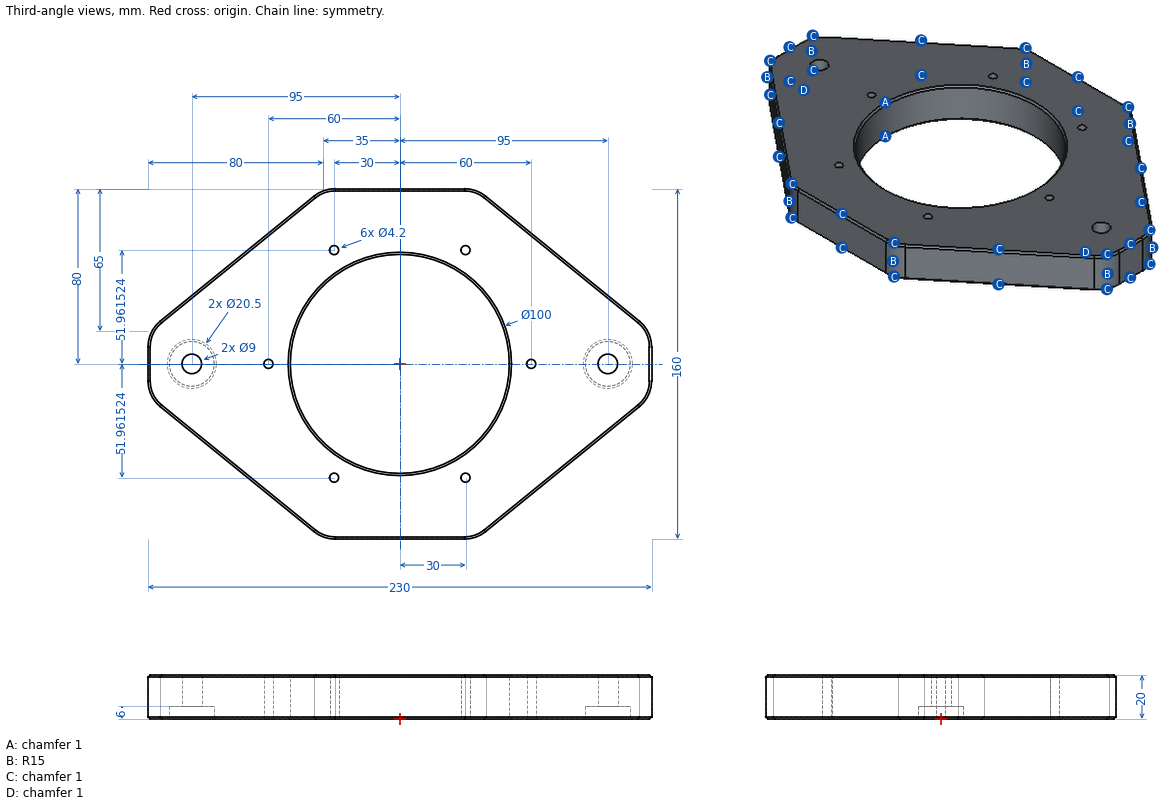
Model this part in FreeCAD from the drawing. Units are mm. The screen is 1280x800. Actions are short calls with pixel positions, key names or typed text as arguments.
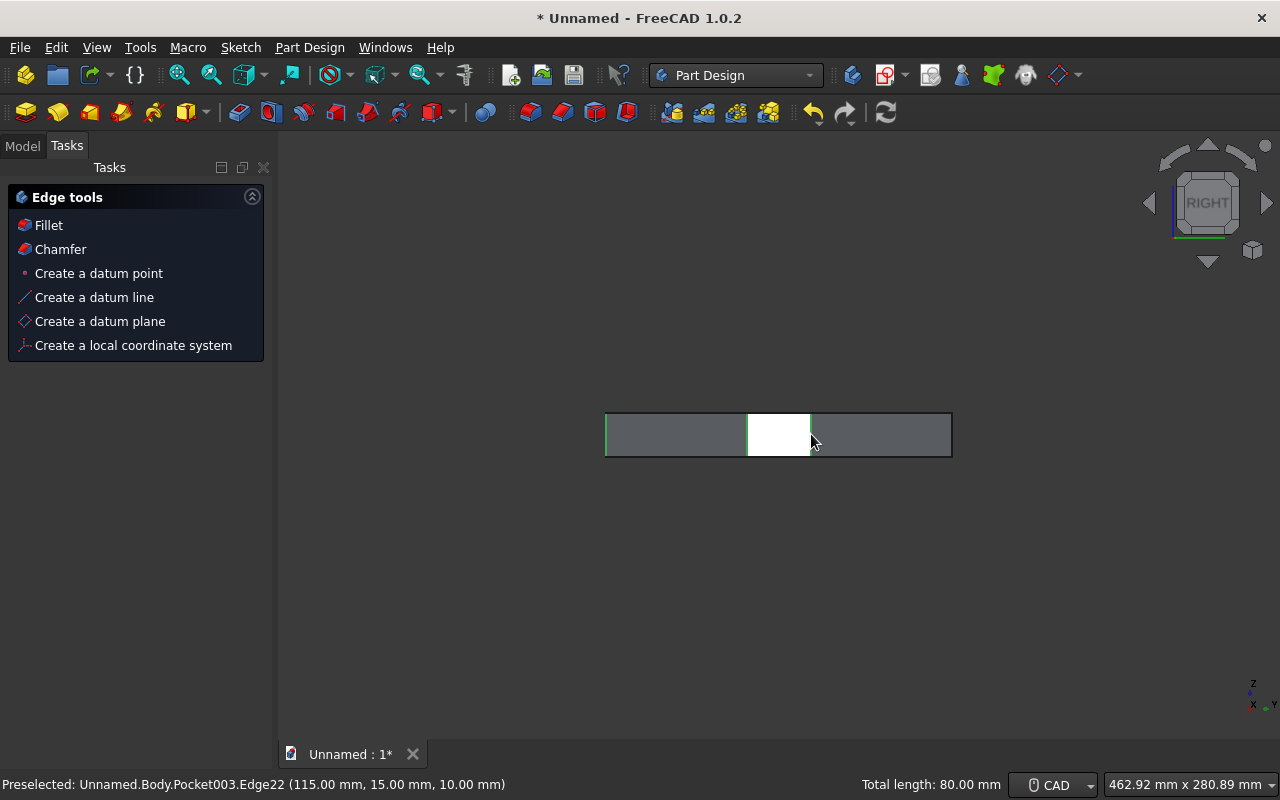
key(5)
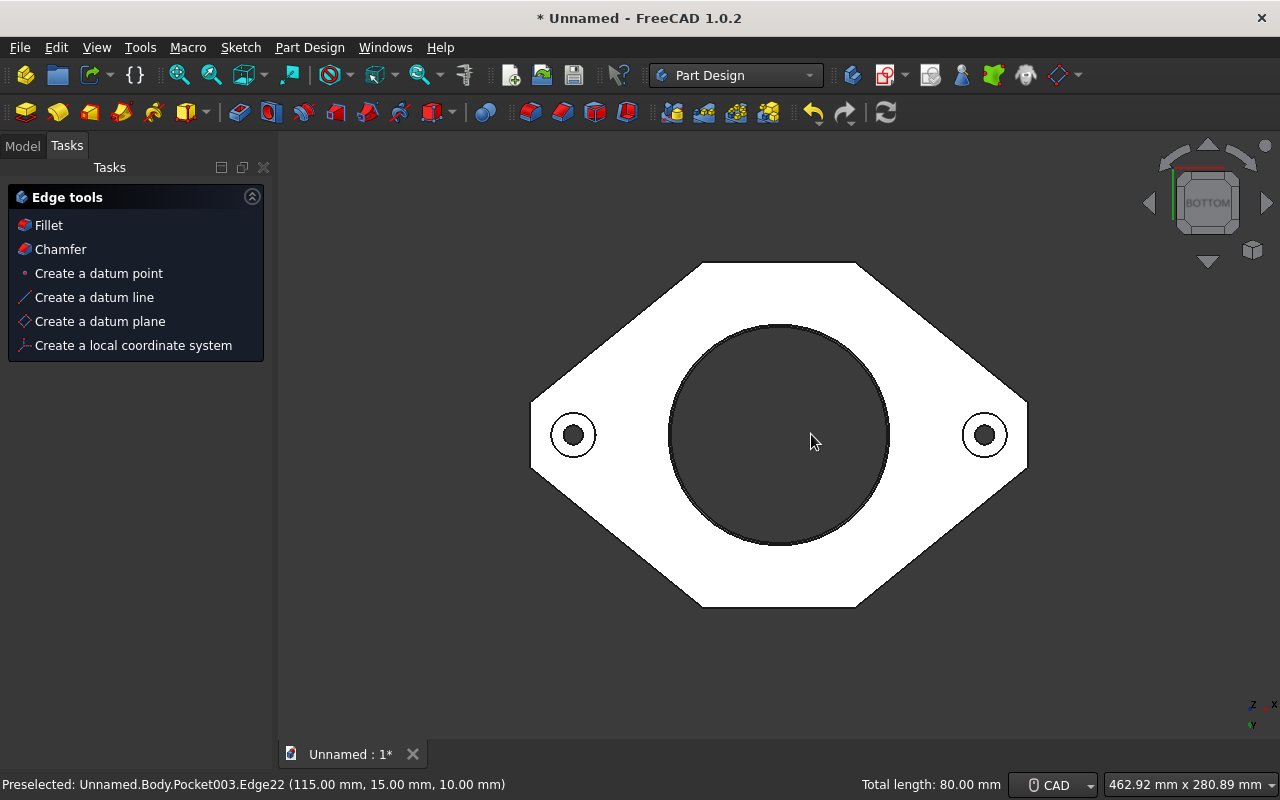
key(4)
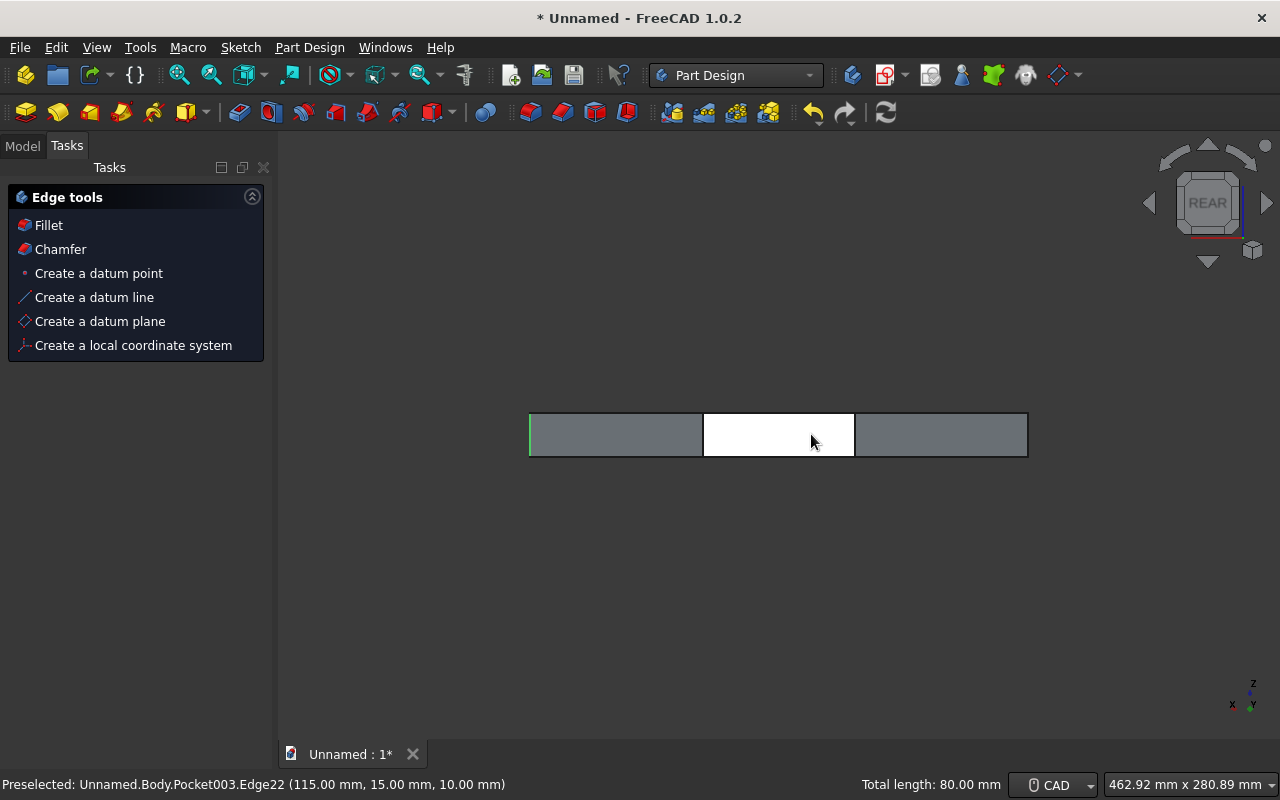
click(703, 434, ctrl)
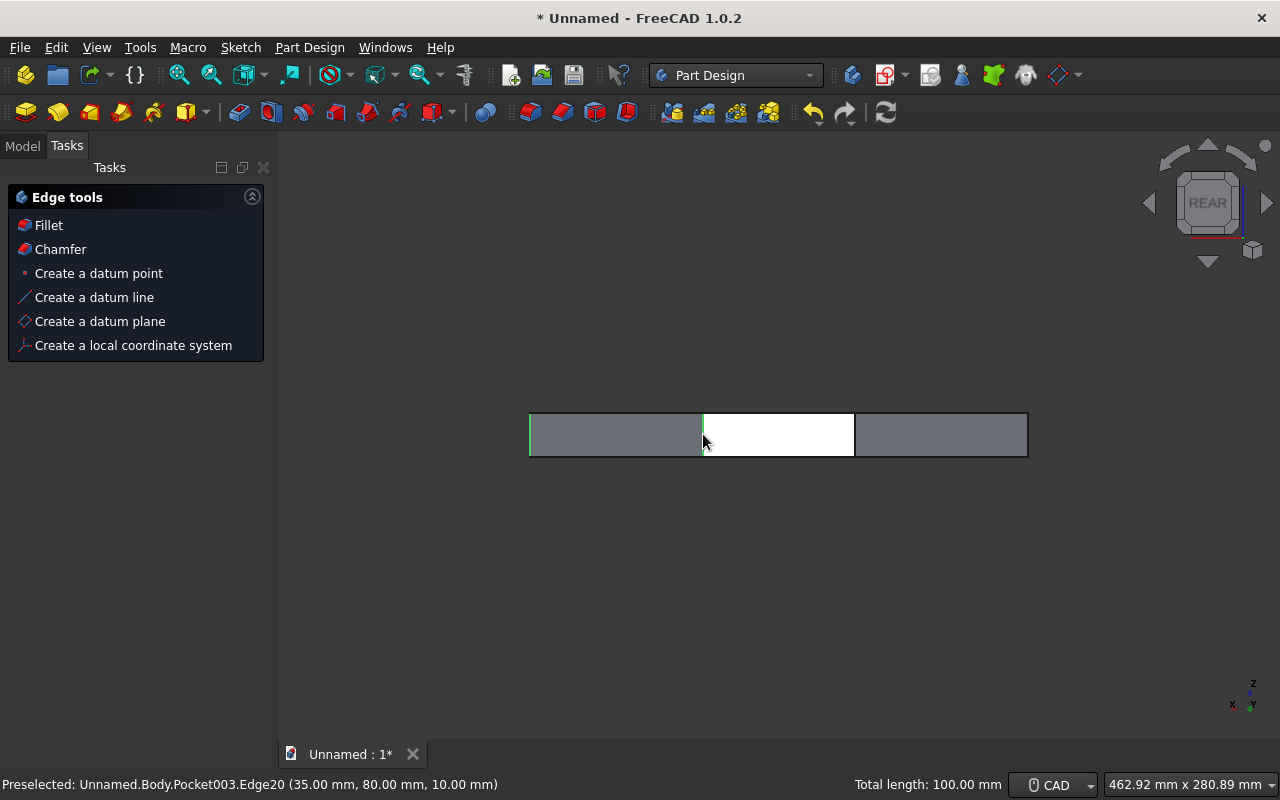
click(855, 434, ctrl)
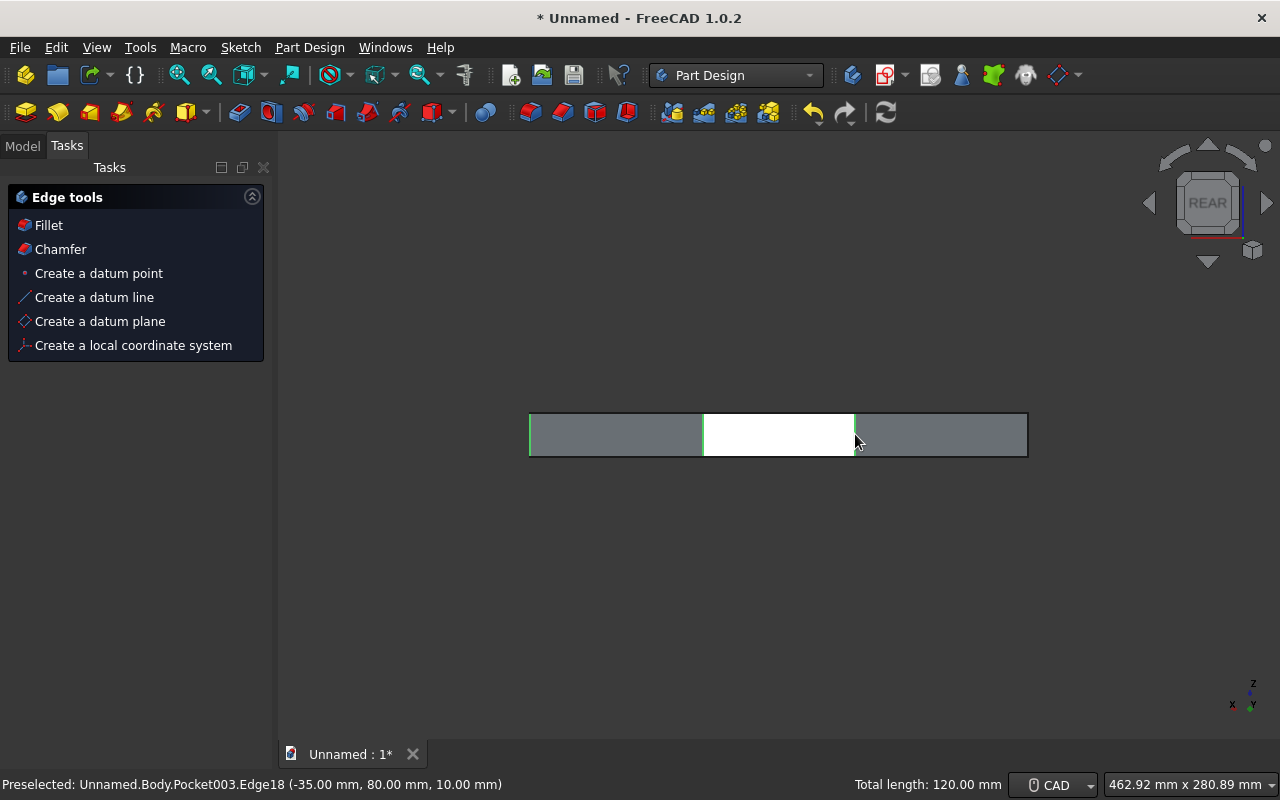
key(6)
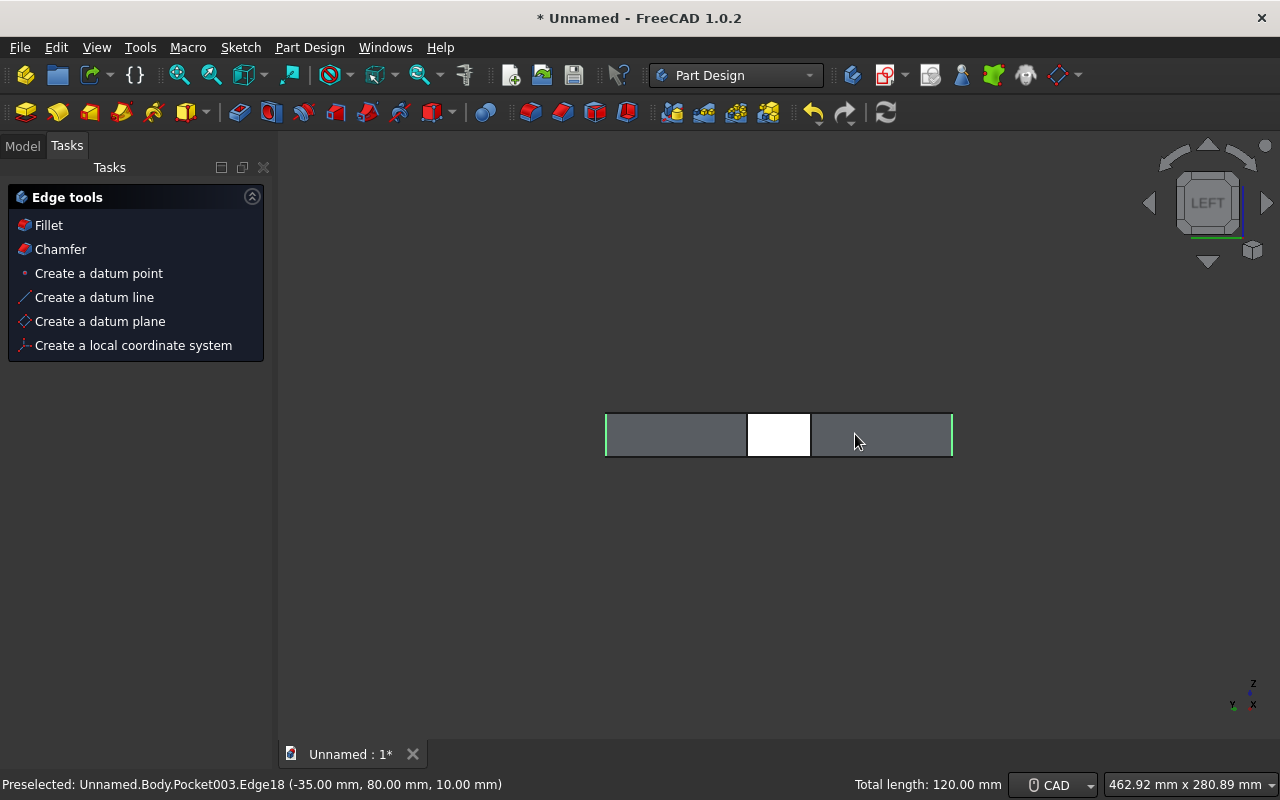
click(180, 76)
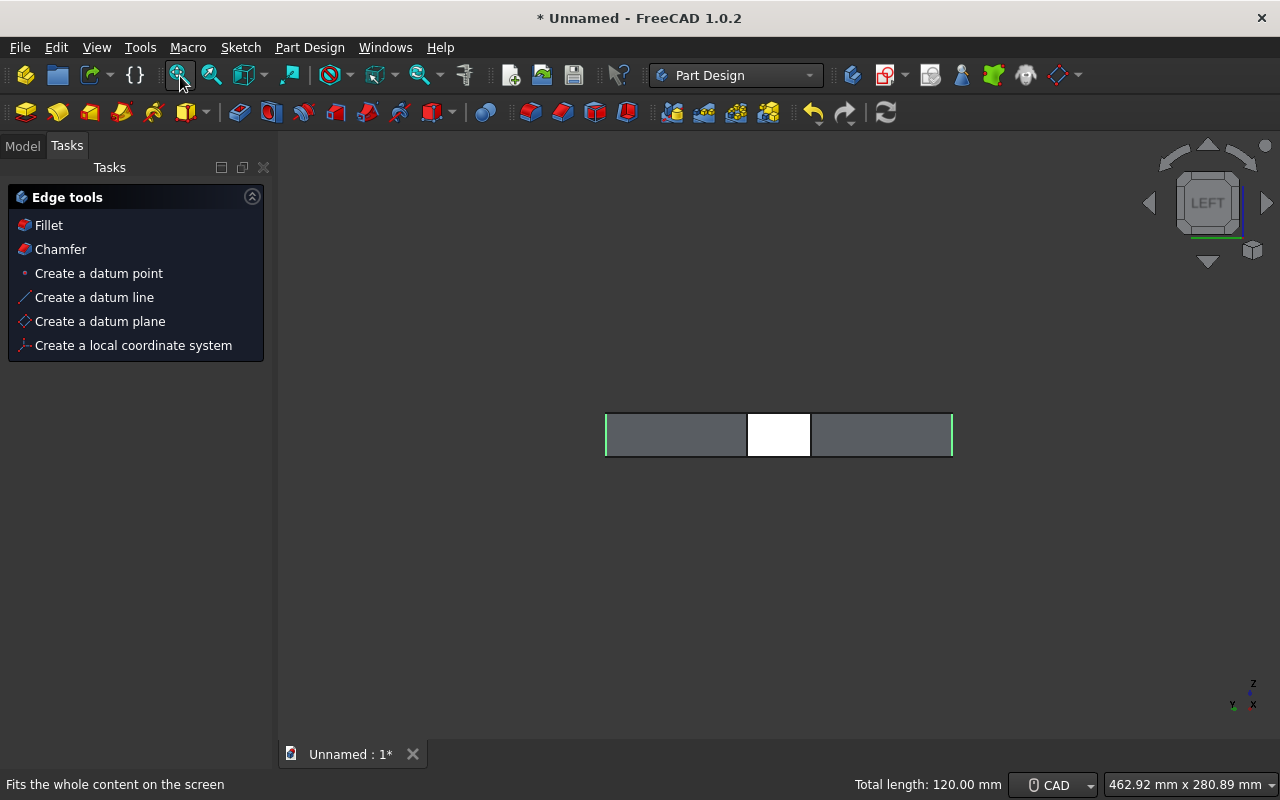
click(811, 434, ctrl)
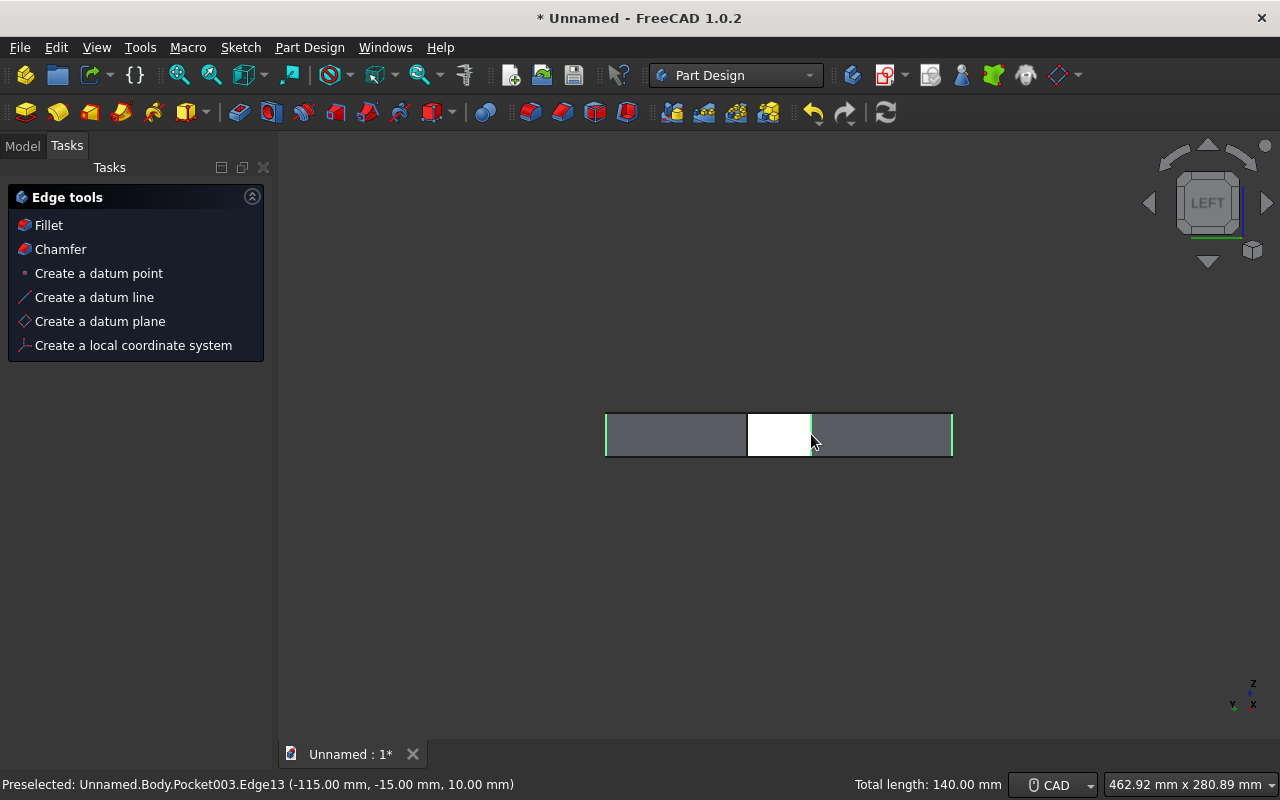
click(747, 434, ctrl)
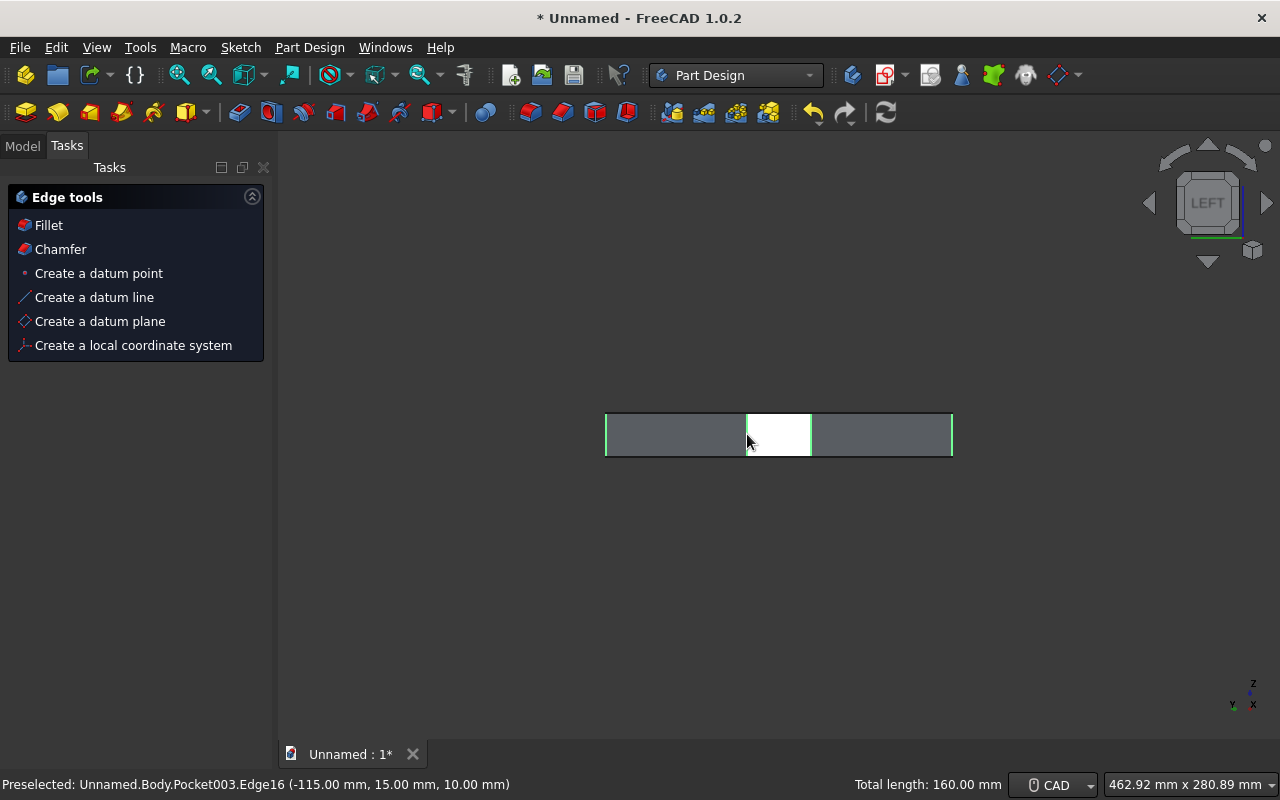
click(532, 112)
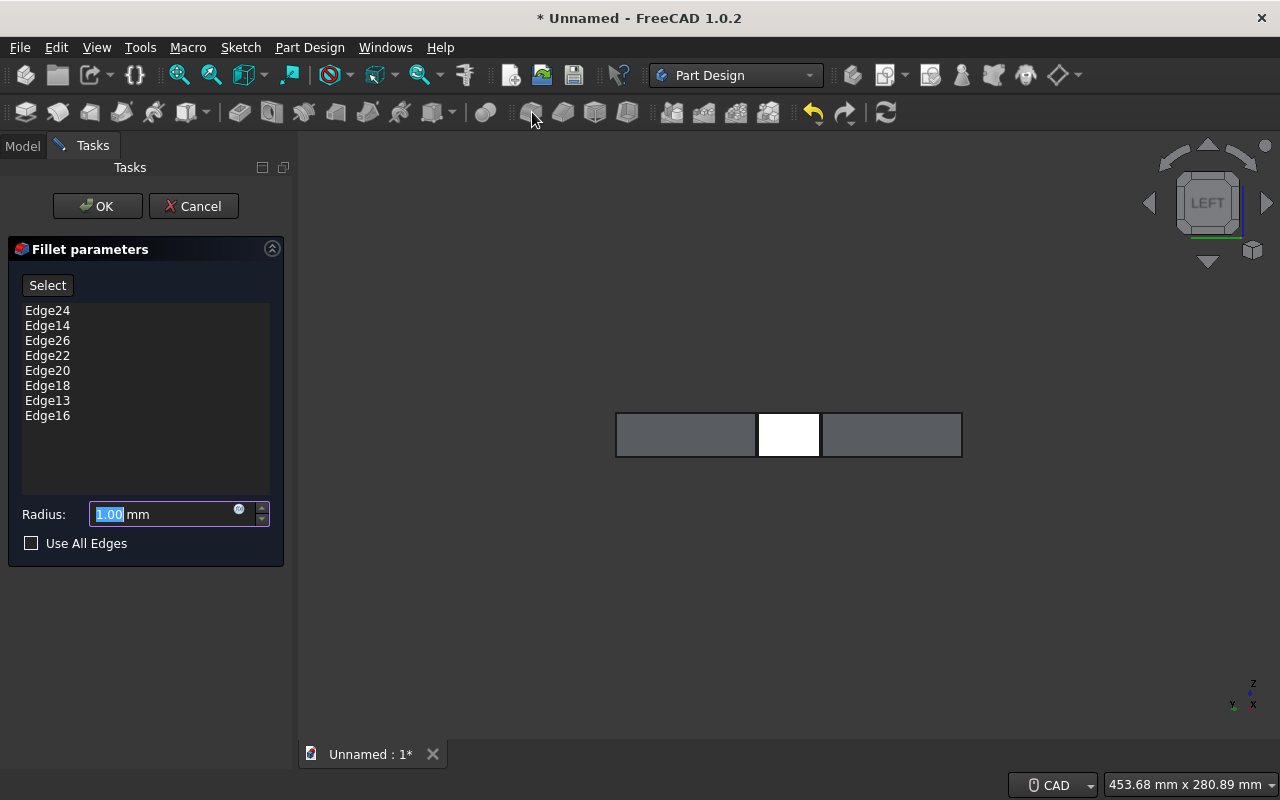
text(15)
key(Tab)